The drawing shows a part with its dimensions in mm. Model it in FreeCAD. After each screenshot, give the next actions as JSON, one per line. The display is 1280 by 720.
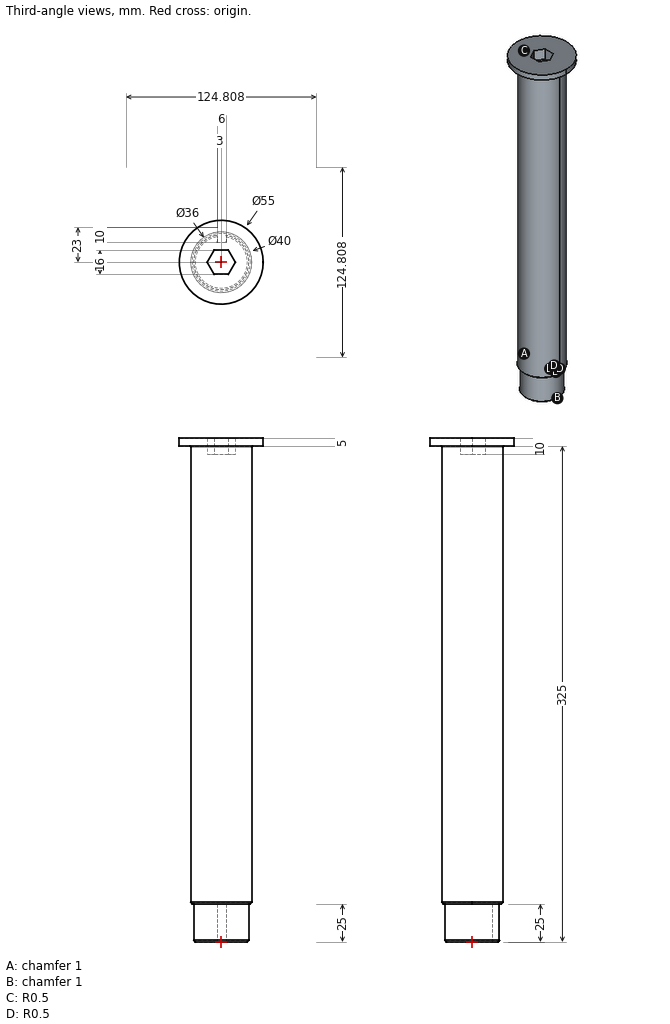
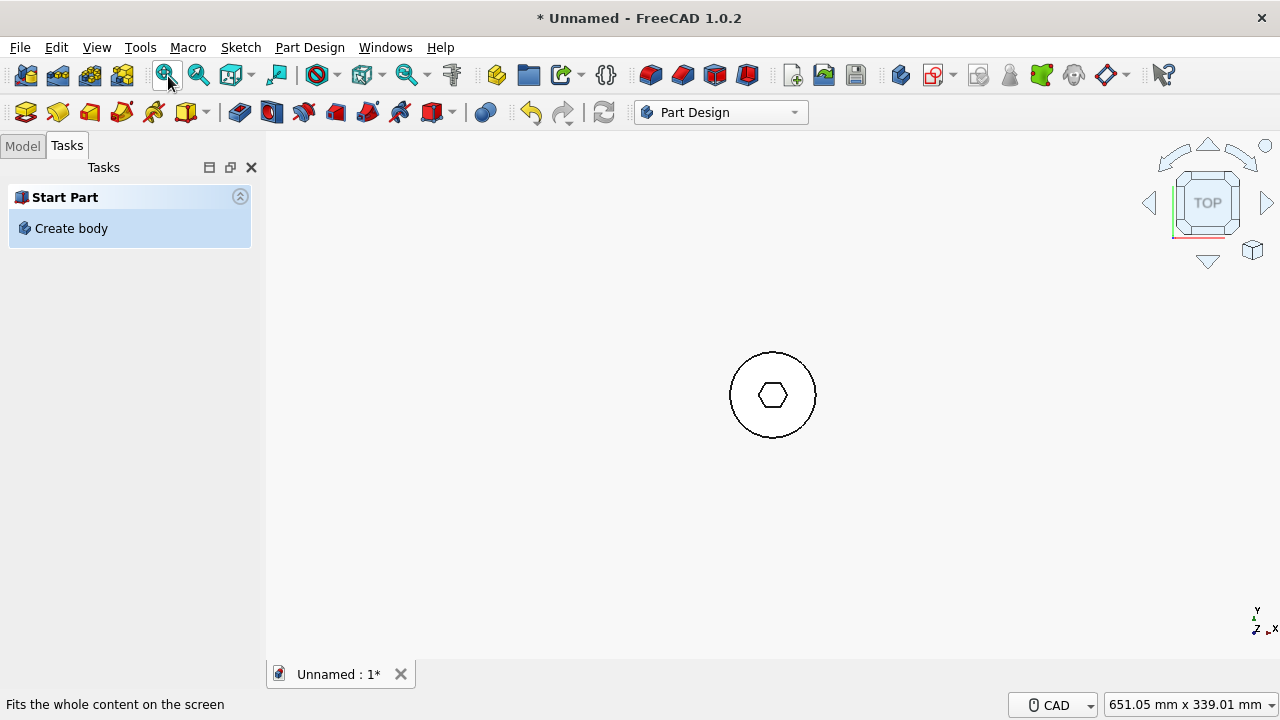
{"action": "key", "text": "0"}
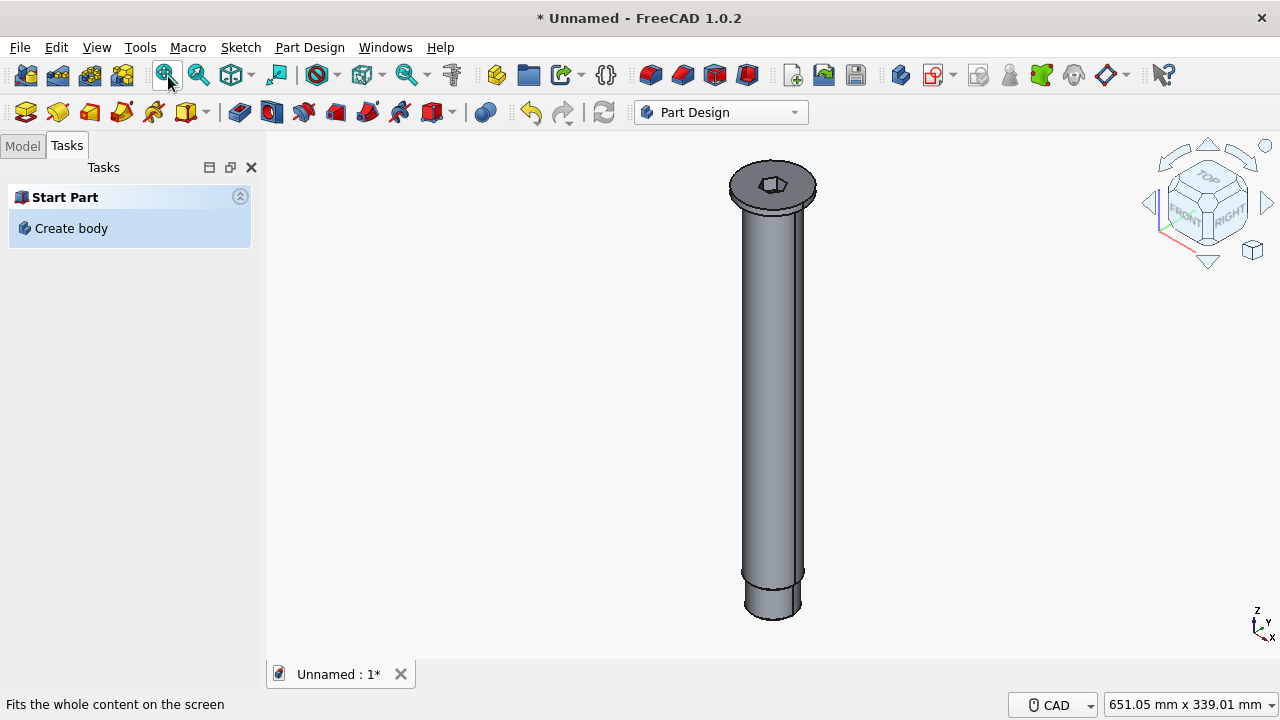
{"action": "key", "text": "1"}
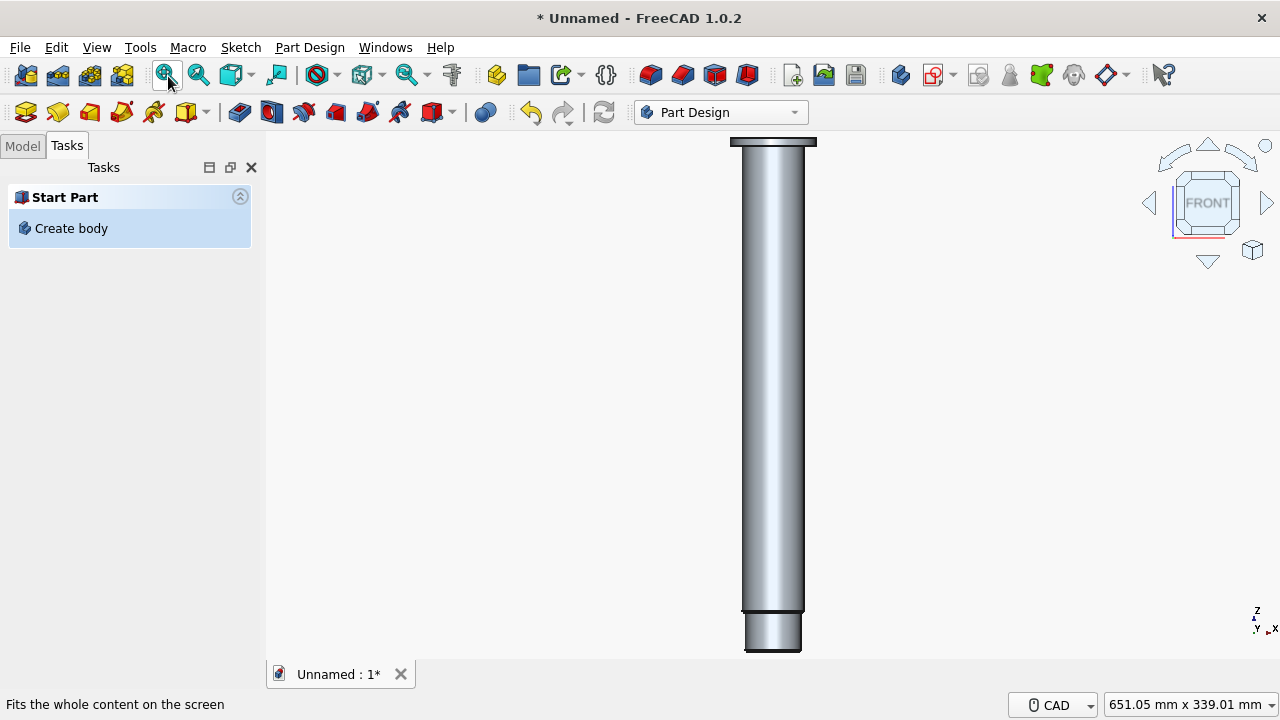
{"action": "key", "text": "3"}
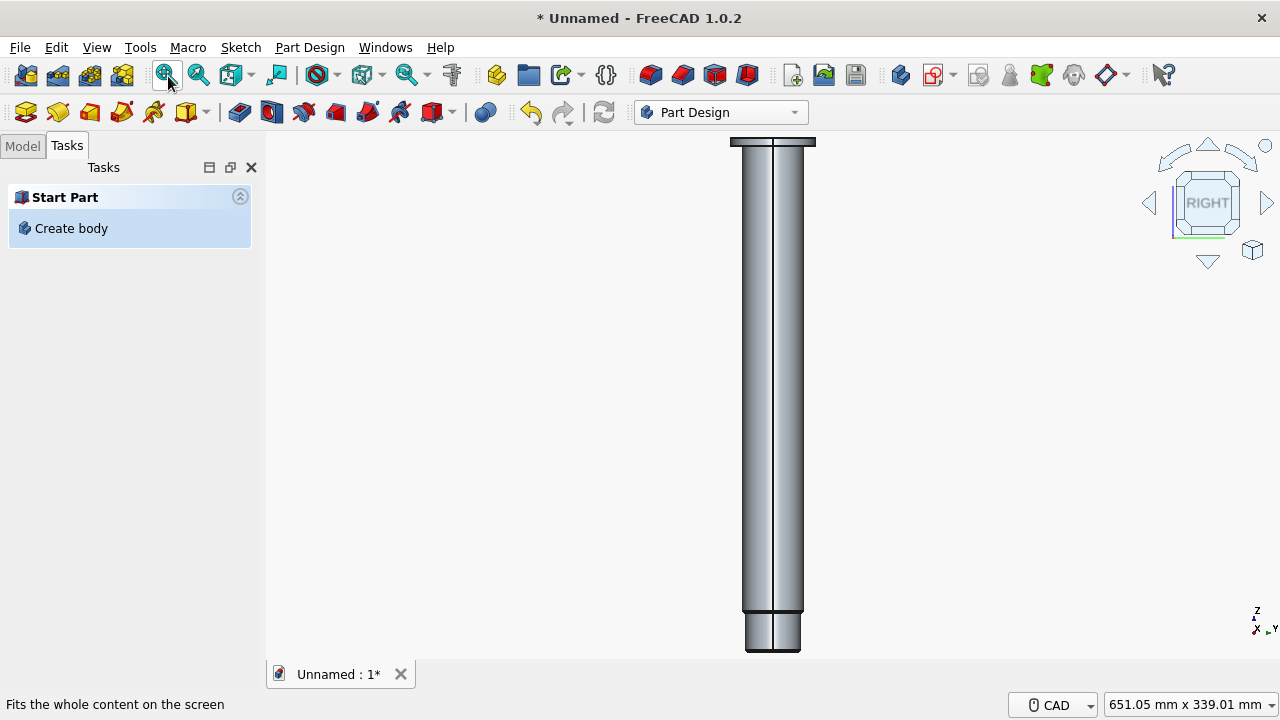
{"action": "key", "text": "5"}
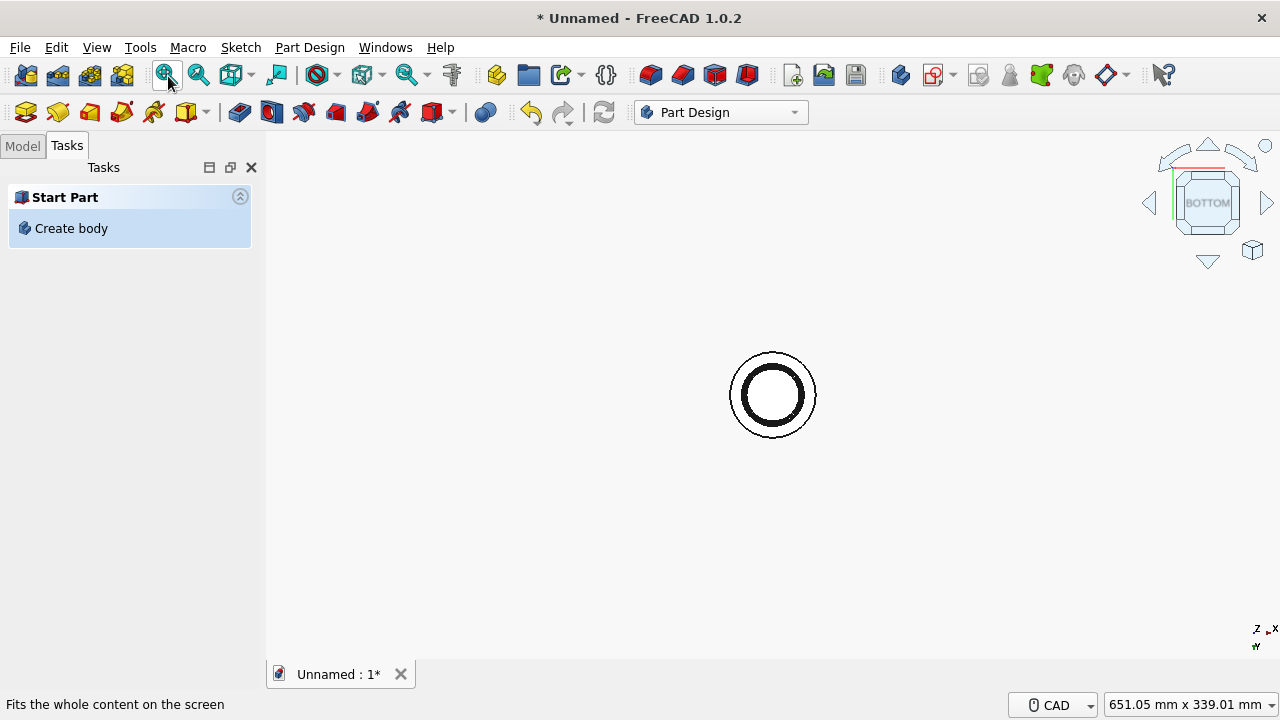
{"action": "left_click", "coordinate": [168, 76]}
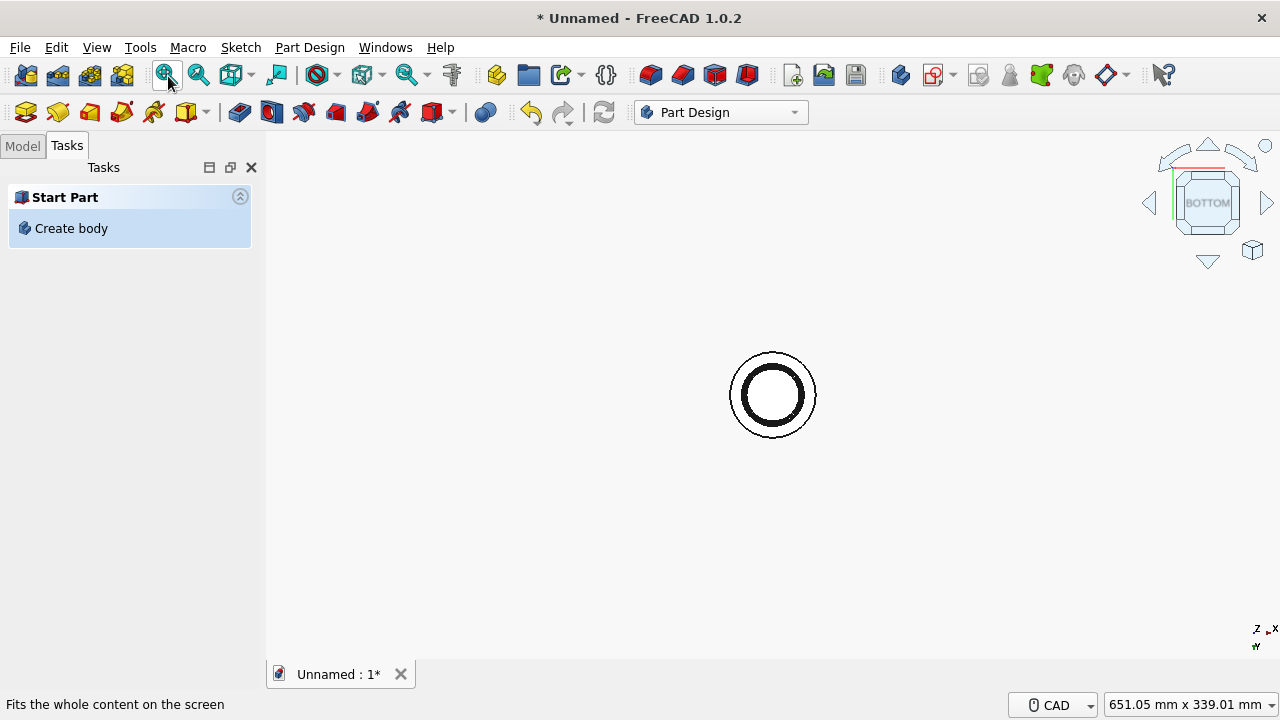
{"action": "key", "text": "4"}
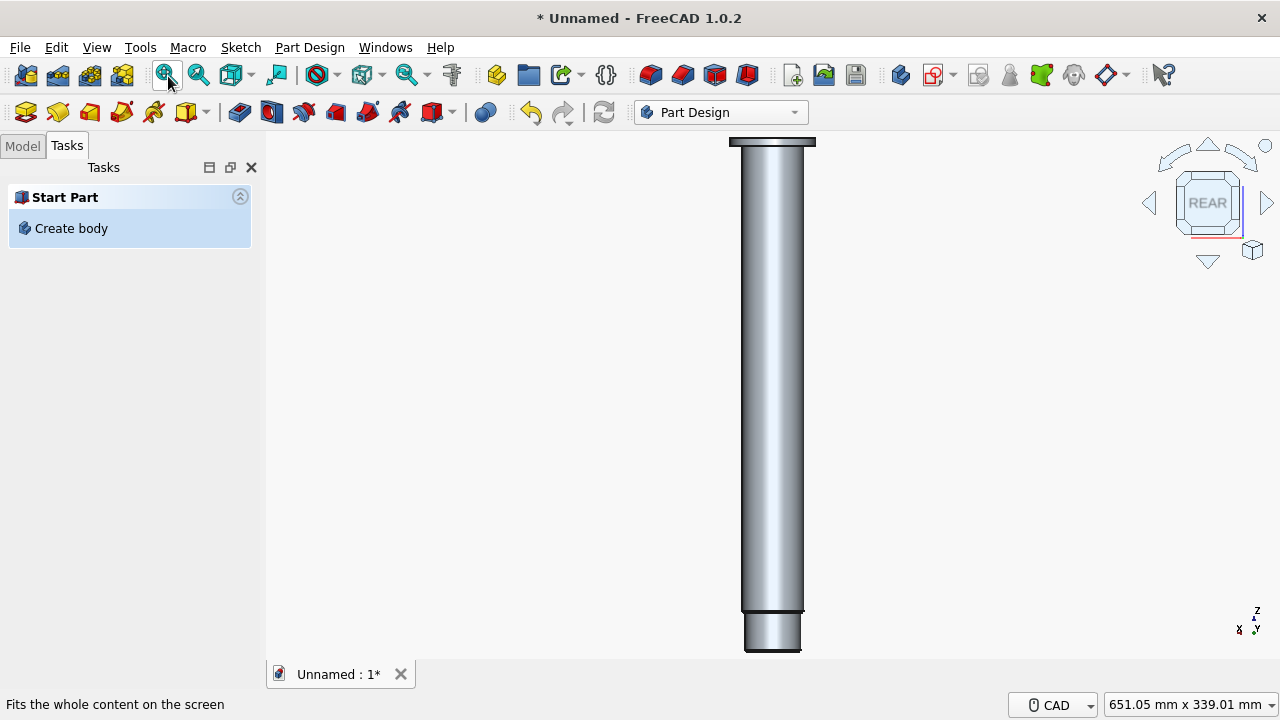
{"action": "key", "text": "6"}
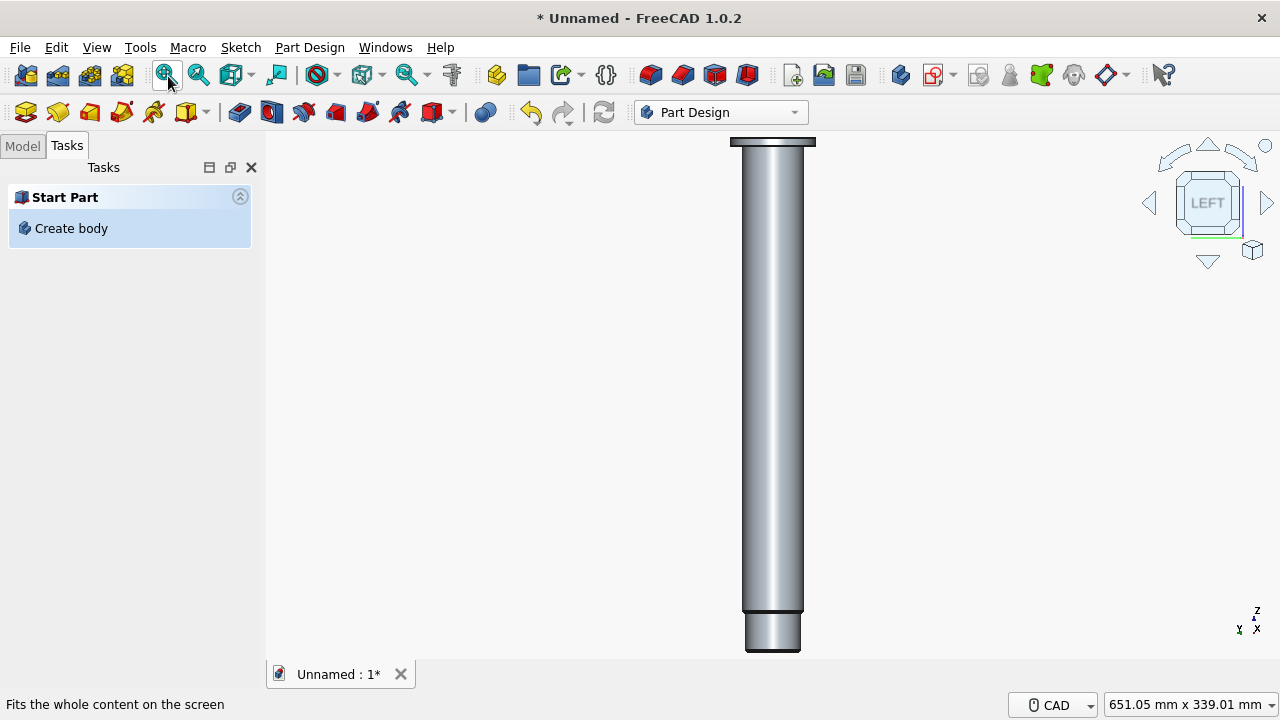
{"action": "key", "text": "v 3"}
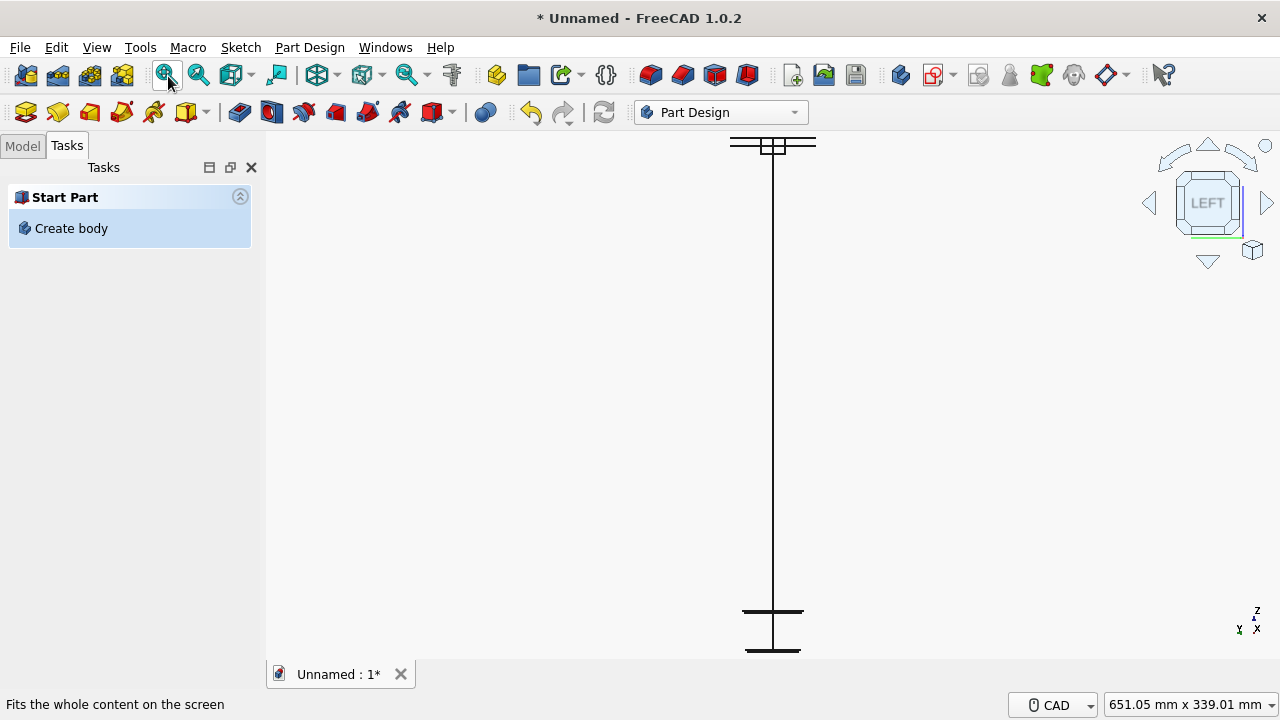
{"action": "key", "text": "0"}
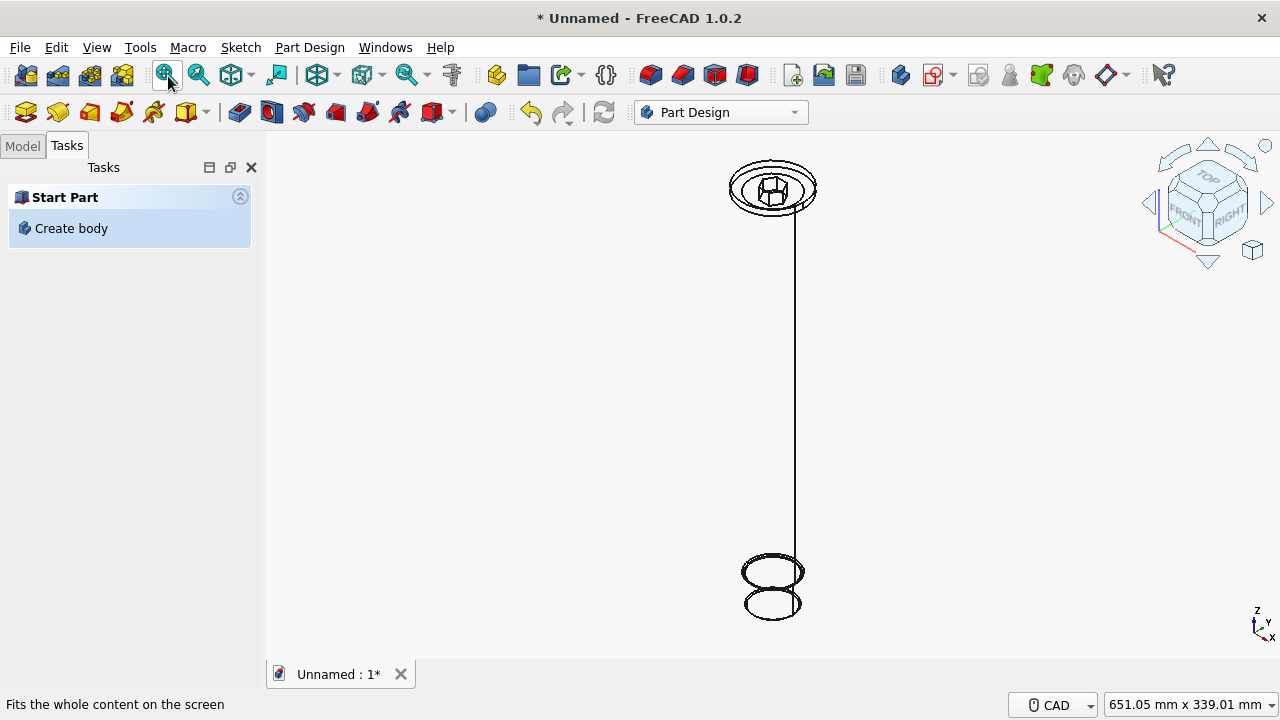
{"action": "left_click", "coordinate": [751, 178]}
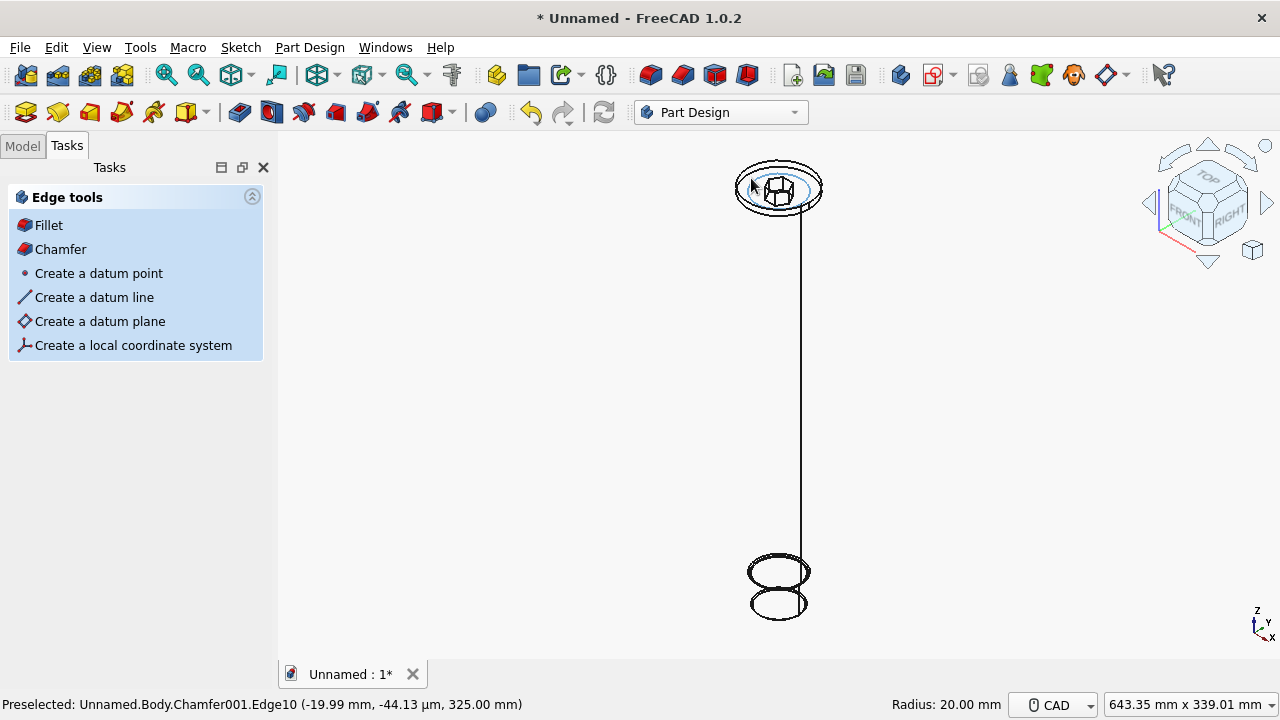
{"action": "key", "text": "v 1"}